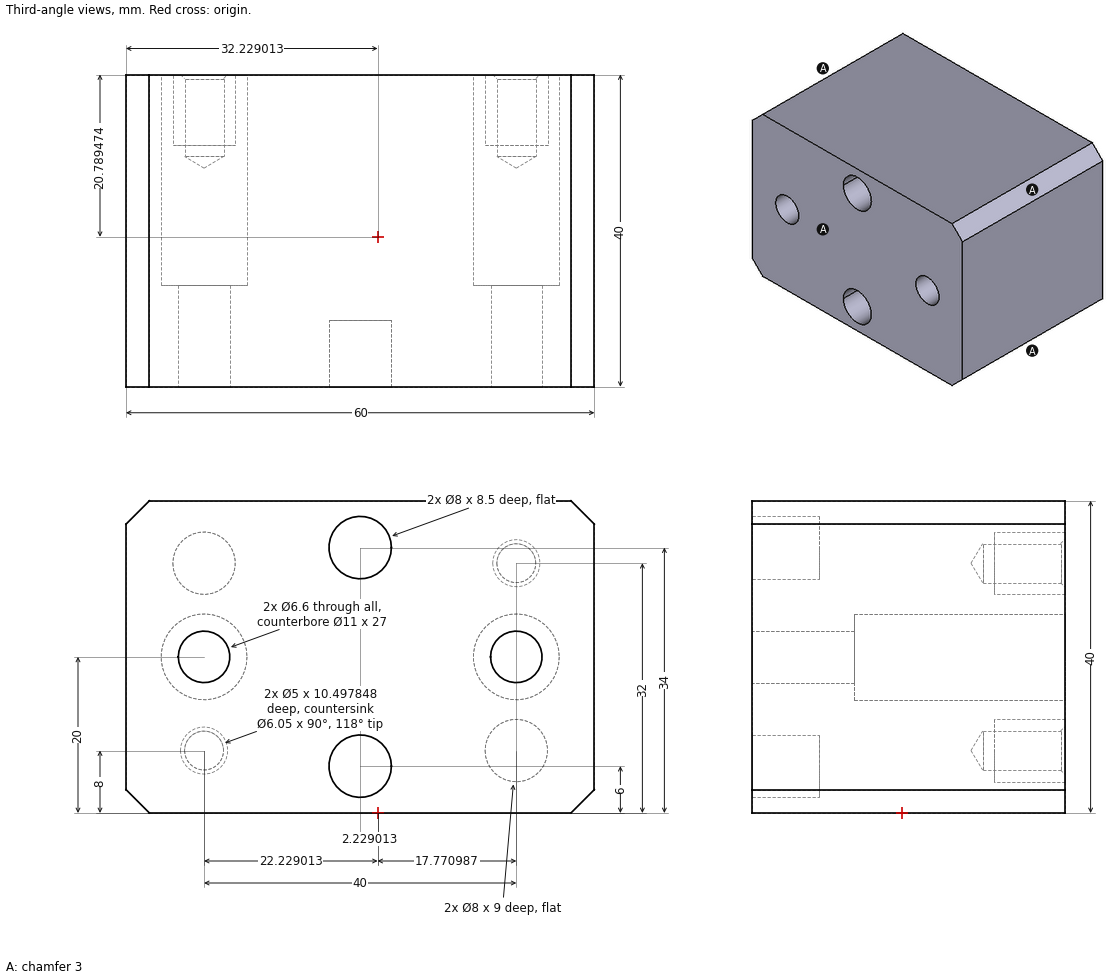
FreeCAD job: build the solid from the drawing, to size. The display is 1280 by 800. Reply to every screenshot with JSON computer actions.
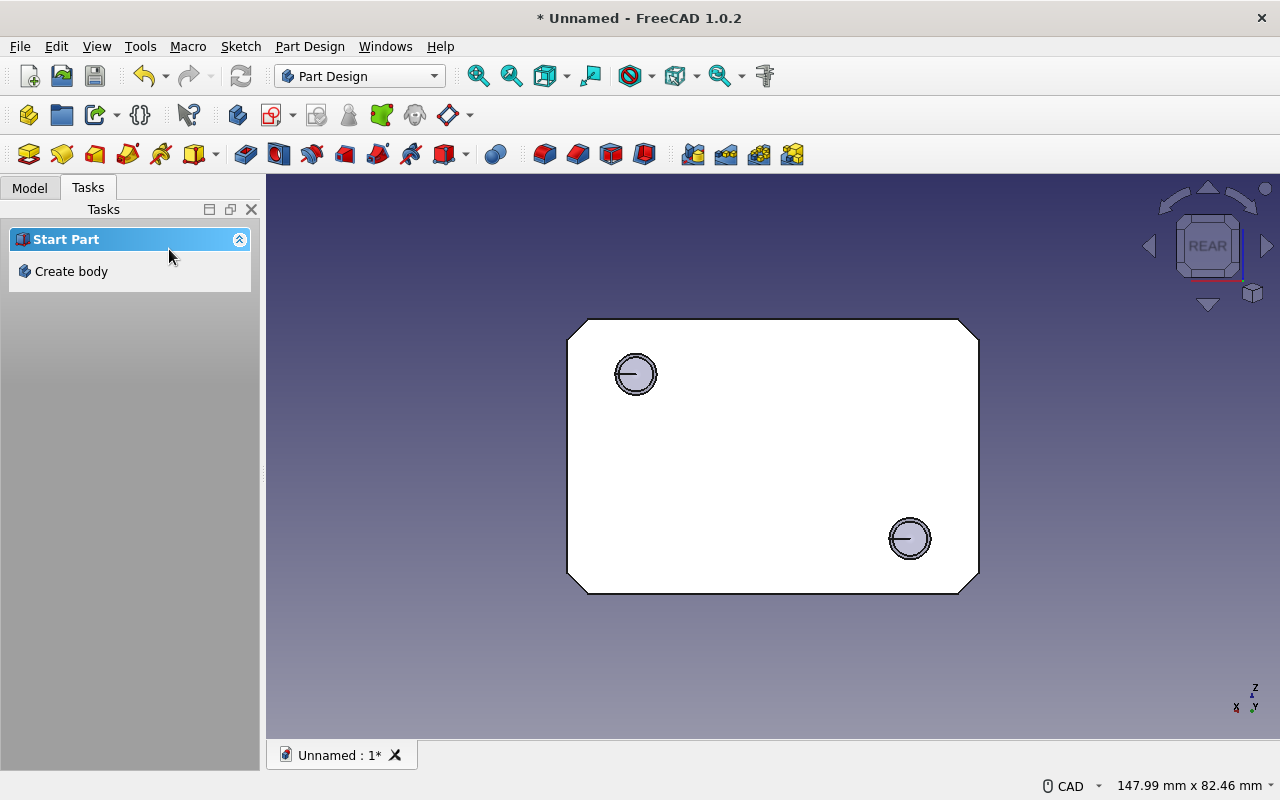
{"action": "left_click", "coordinate": [773, 455]}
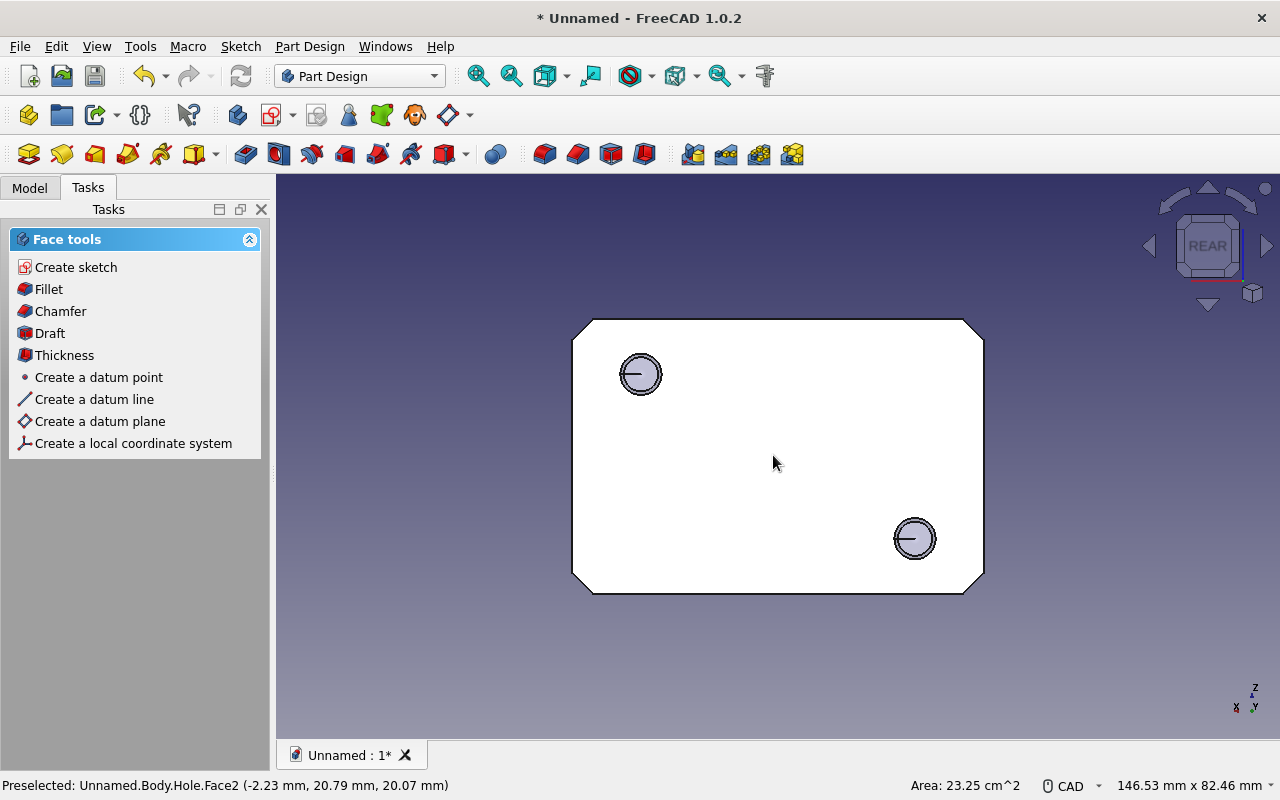
{"action": "left_click", "coordinate": [270, 116]}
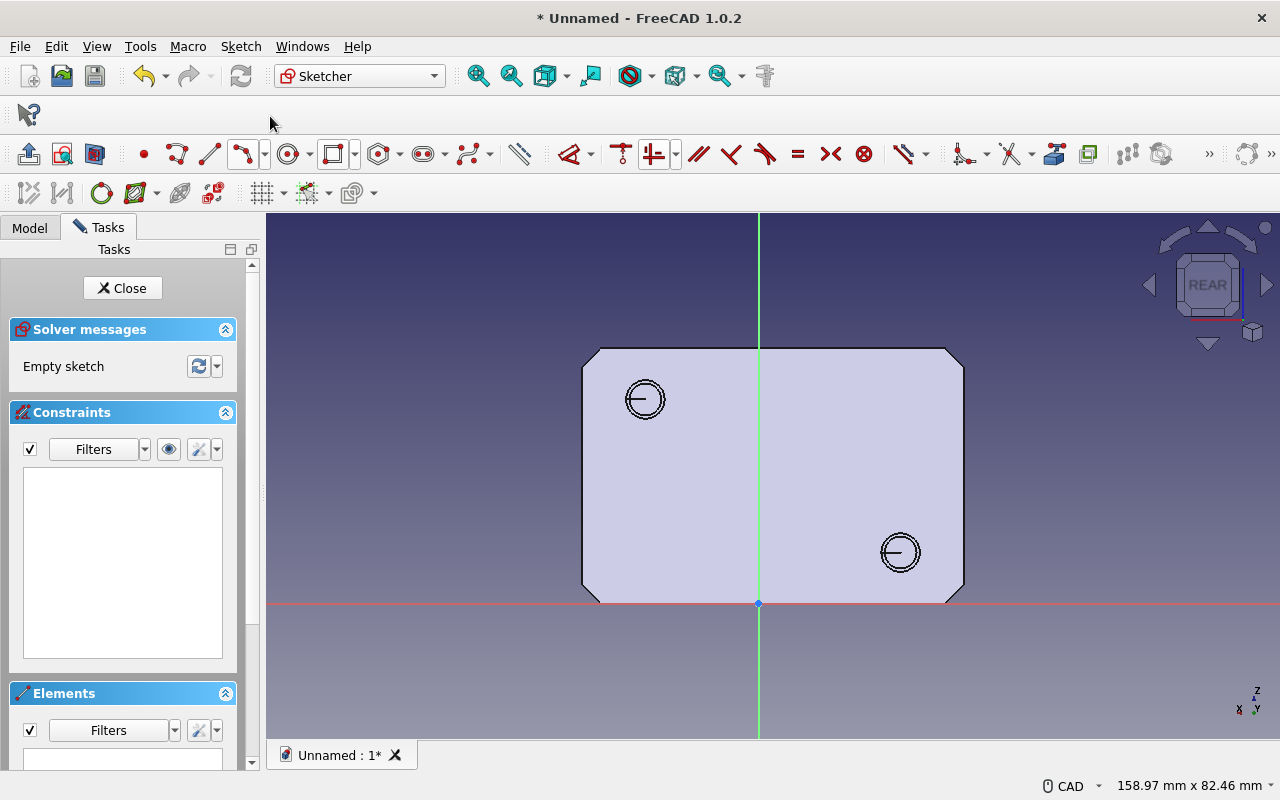
{"action": "scroll", "coordinate": [856, 594], "scroll_direction": "up", "scroll_amount": 3}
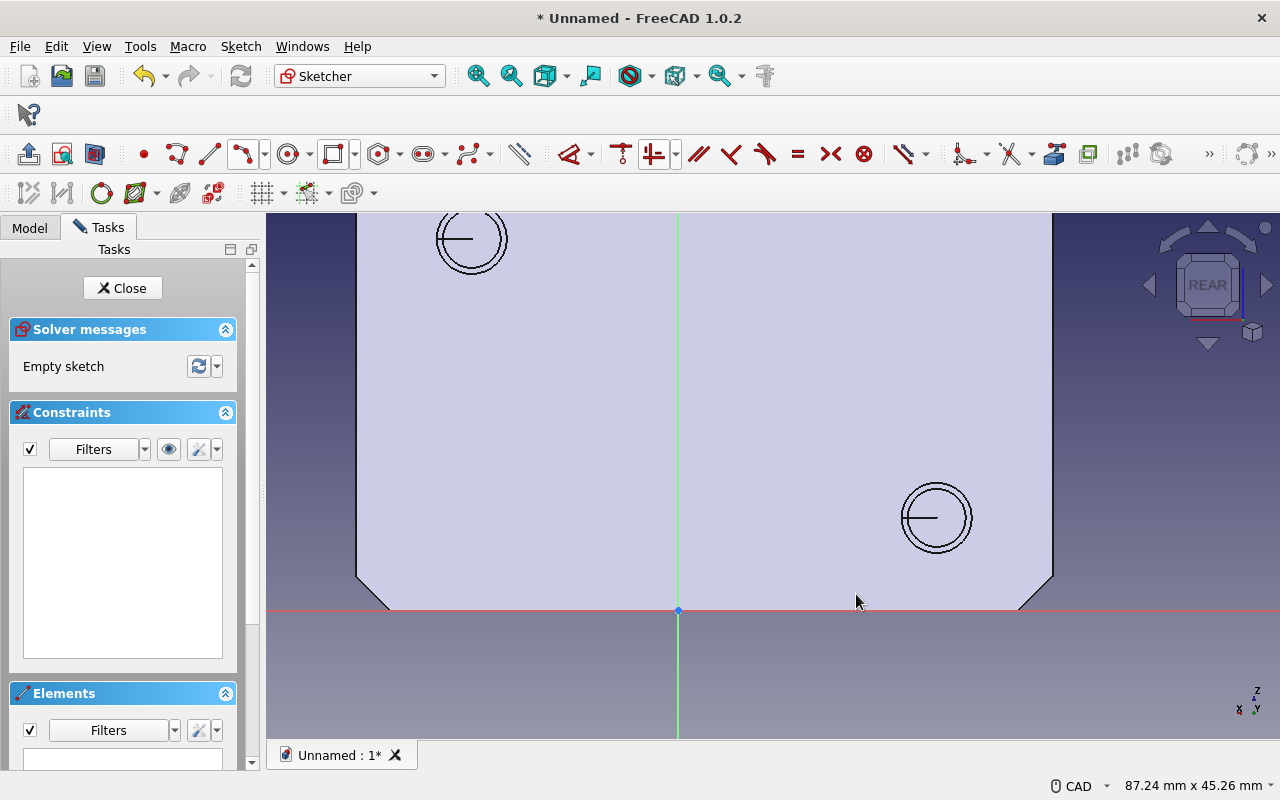
{"action": "key", "text": "g c"}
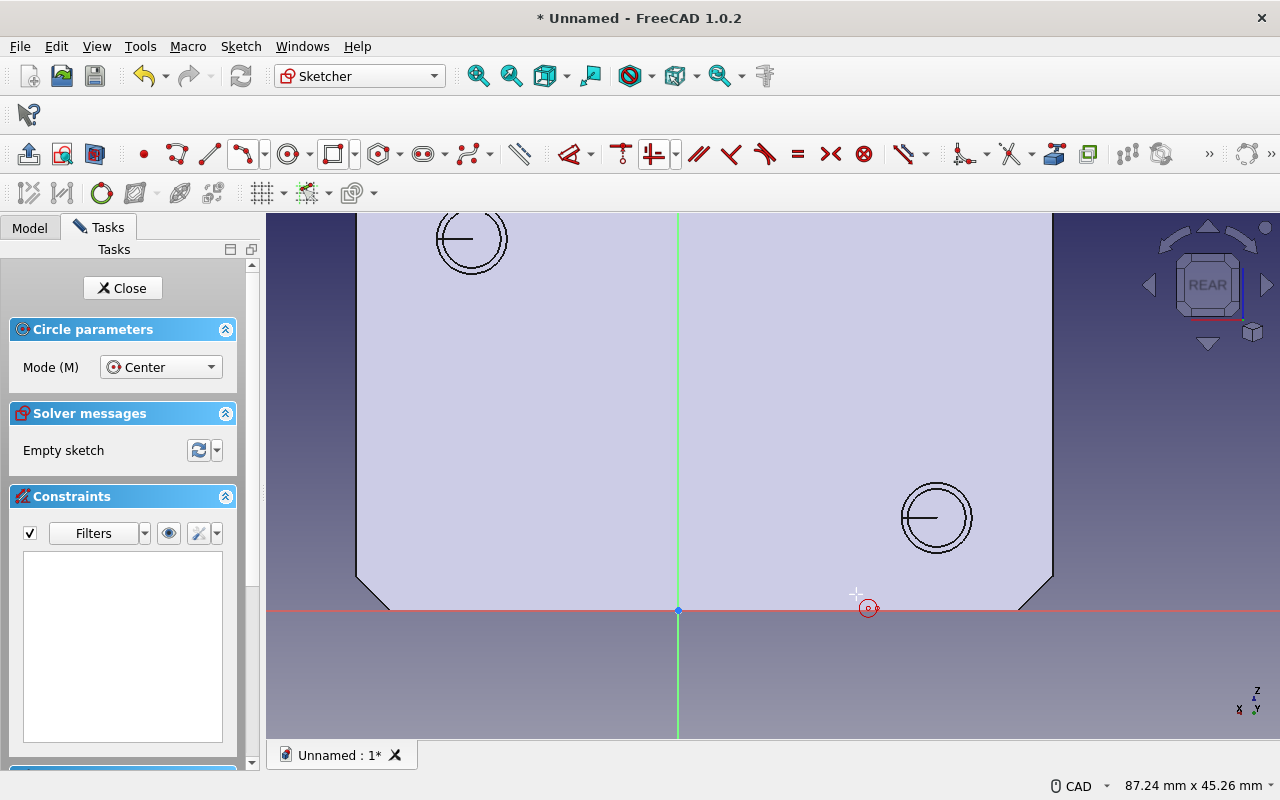
{"action": "left_click", "coordinate": [937, 378]}
{"action": "mouse_move", "coordinate": [964, 351]}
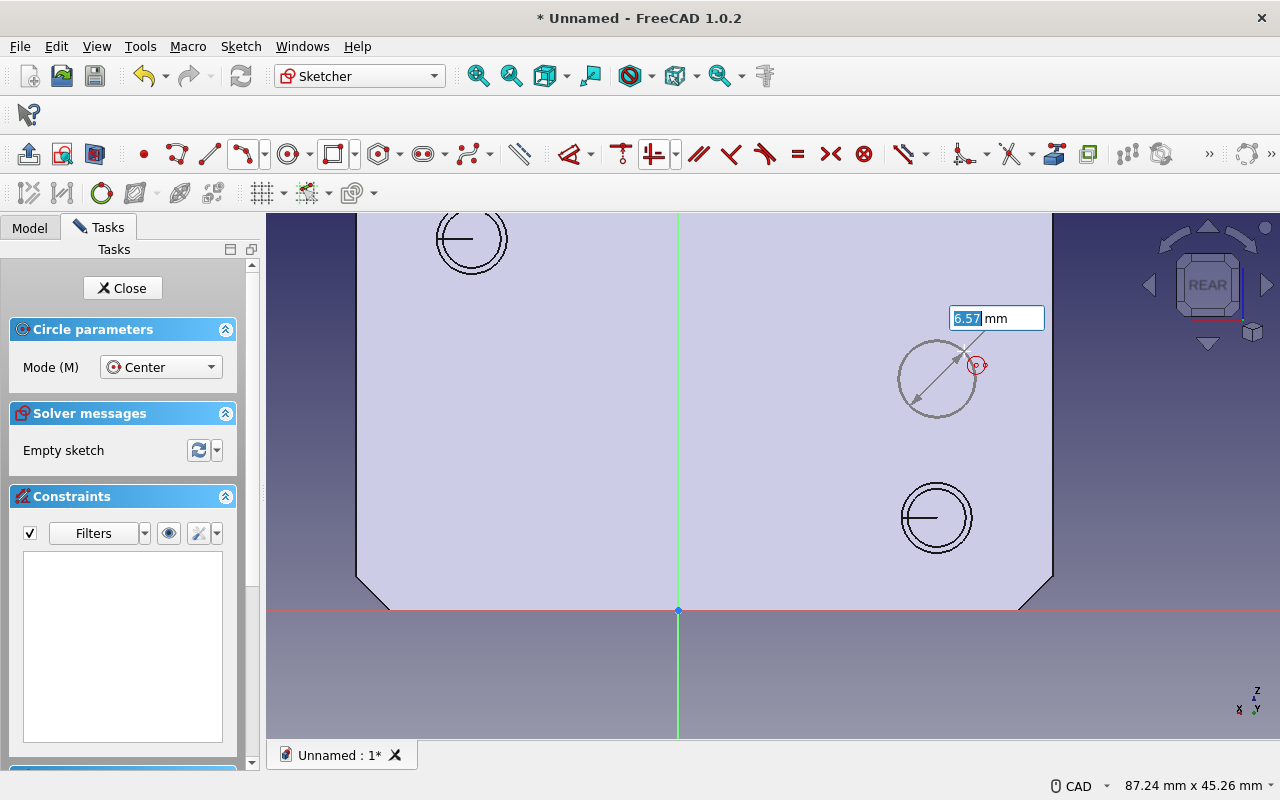
{"action": "type", "text": "6.6"}
{"action": "key", "text": "Return"}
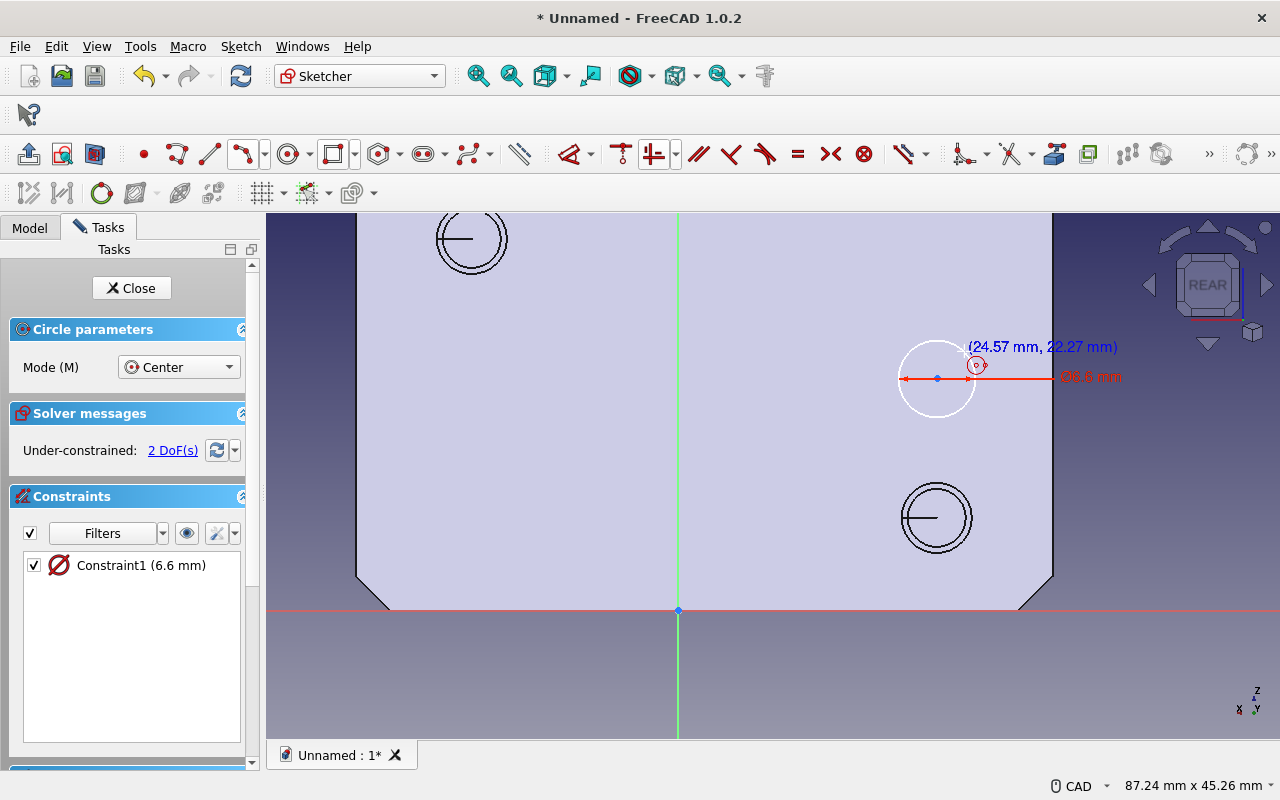
{"action": "left_click", "coordinate": [472, 378]}
{"action": "mouse_move", "coordinate": [499, 351]}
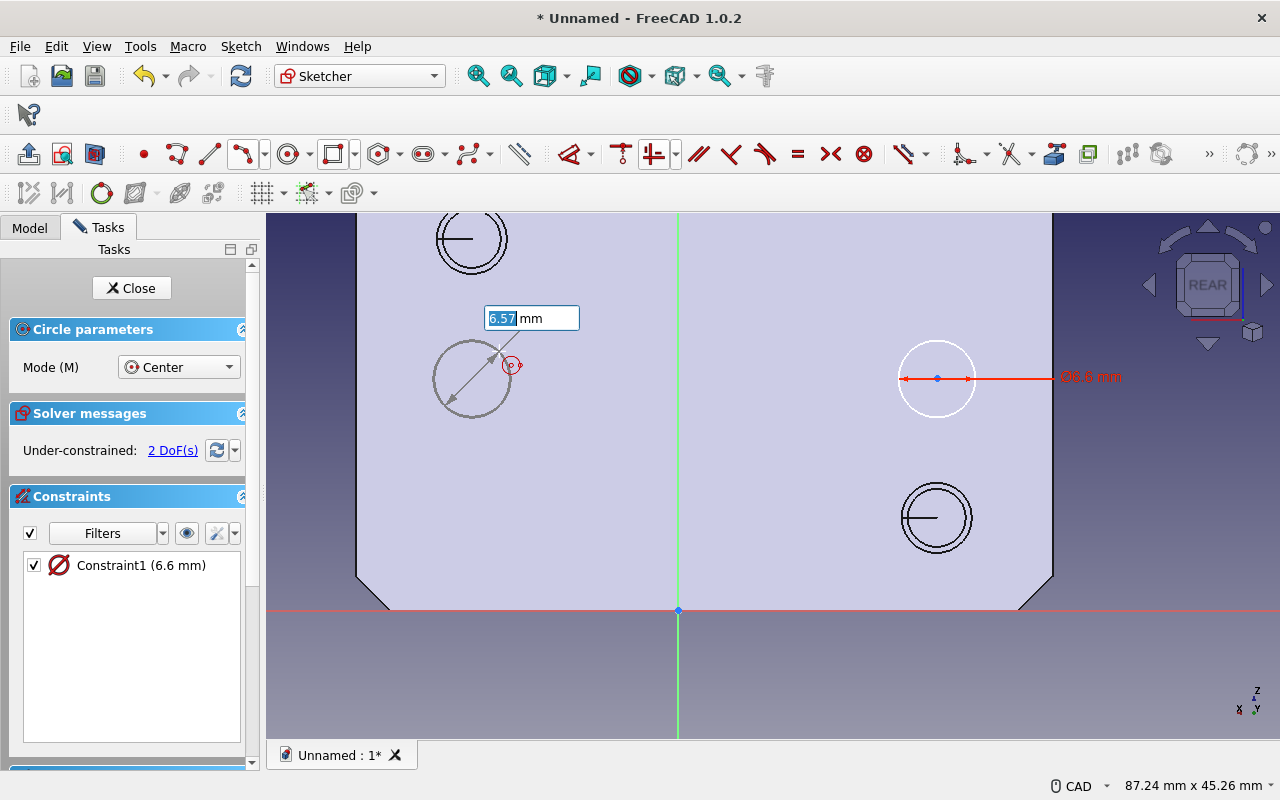
{"action": "type", "text": "6.6"}
{"action": "key", "text": "Return"}
{"action": "key", "text": "Escape"}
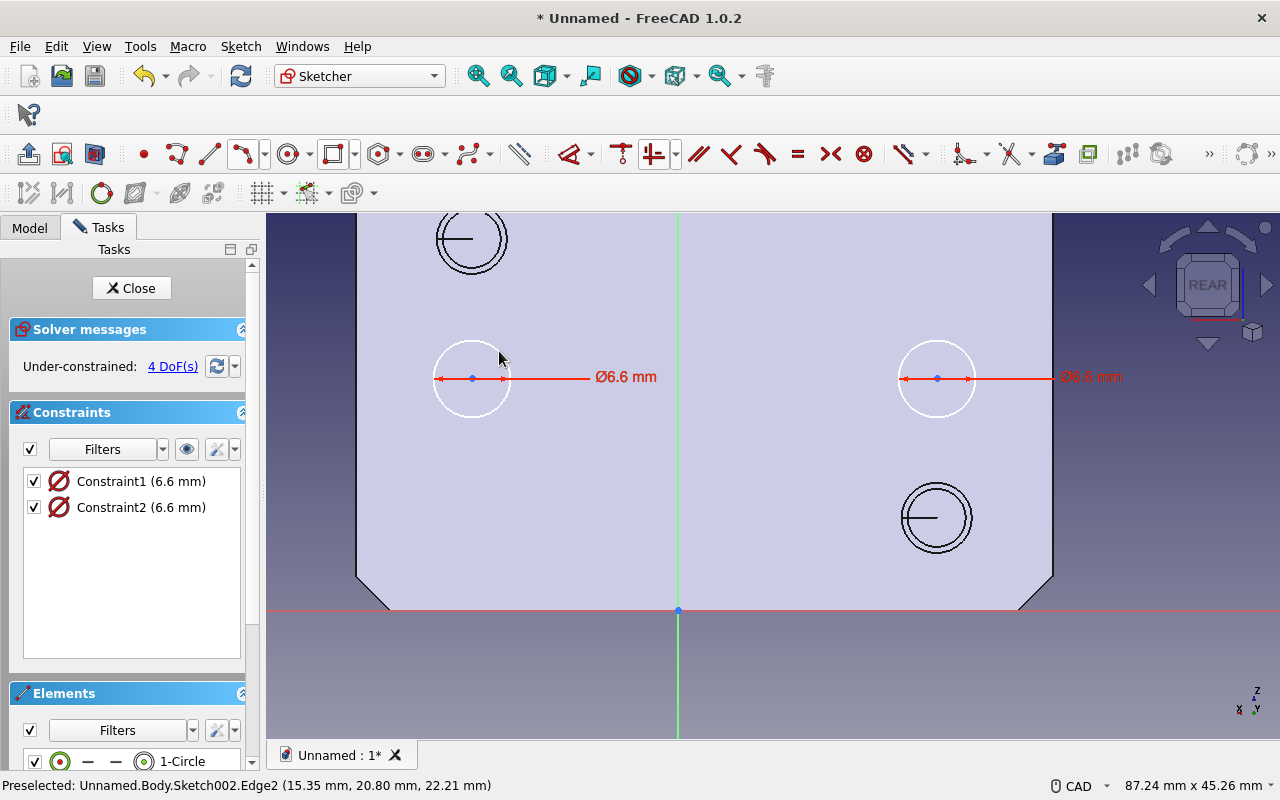
{"action": "left_click", "coordinate": [568, 154]}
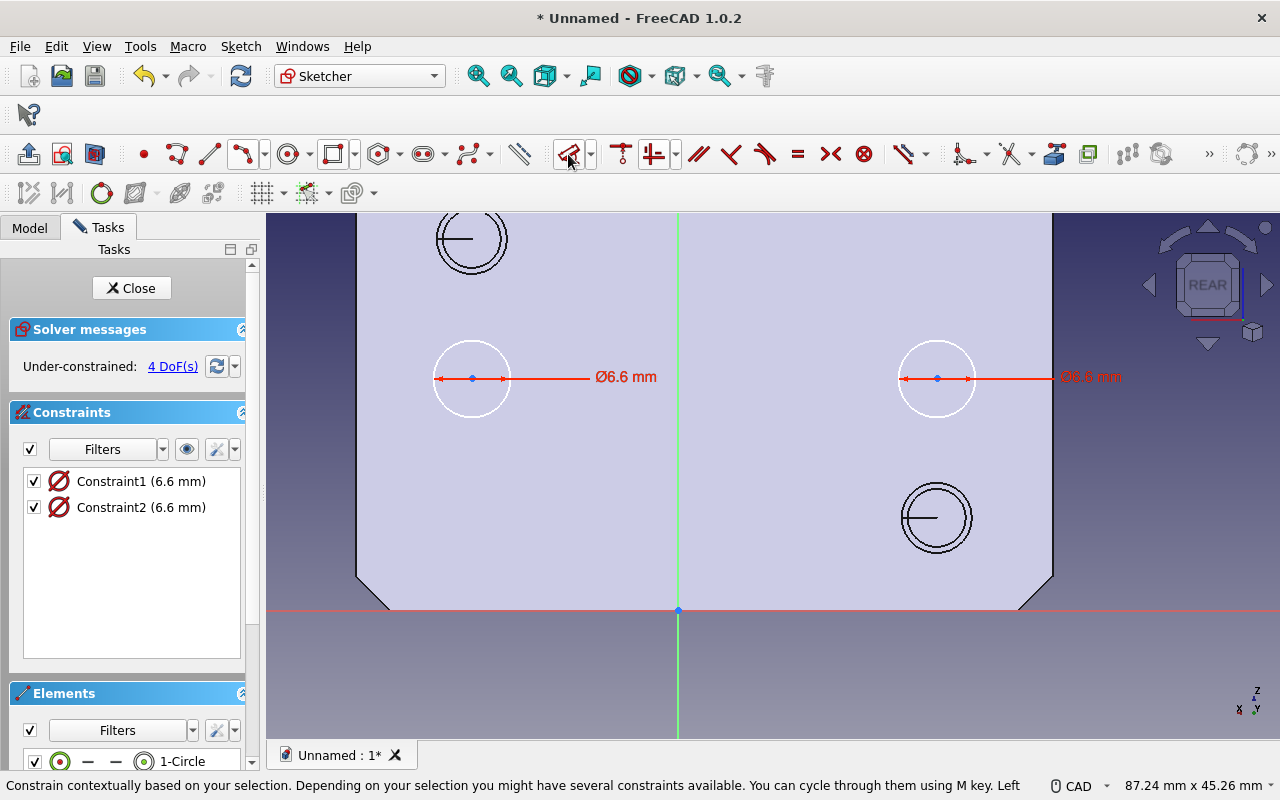
{"action": "left_click", "coordinate": [937, 379]}
{"action": "left_click", "coordinate": [971, 495]}